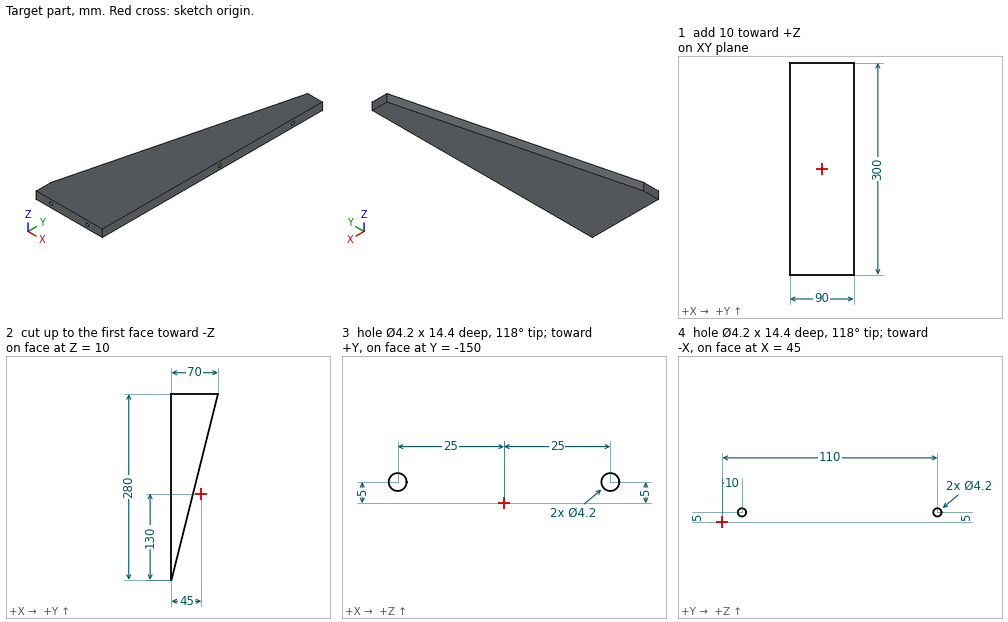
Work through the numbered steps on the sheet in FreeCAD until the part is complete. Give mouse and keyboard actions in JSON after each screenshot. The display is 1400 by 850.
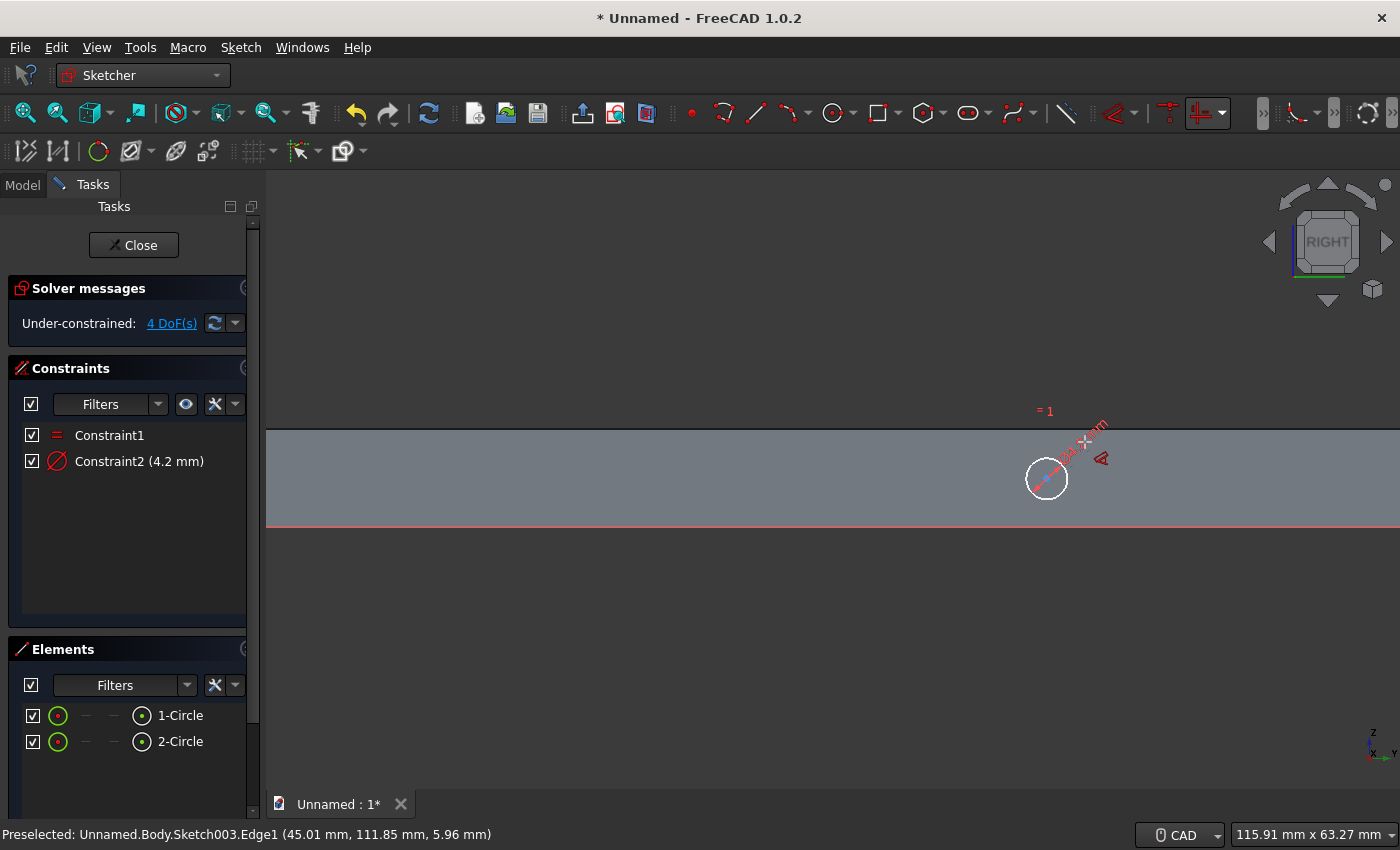
{"action": "left_click", "coordinate": [1047, 479]}
{"action": "left_click", "coordinate": [1081, 503]}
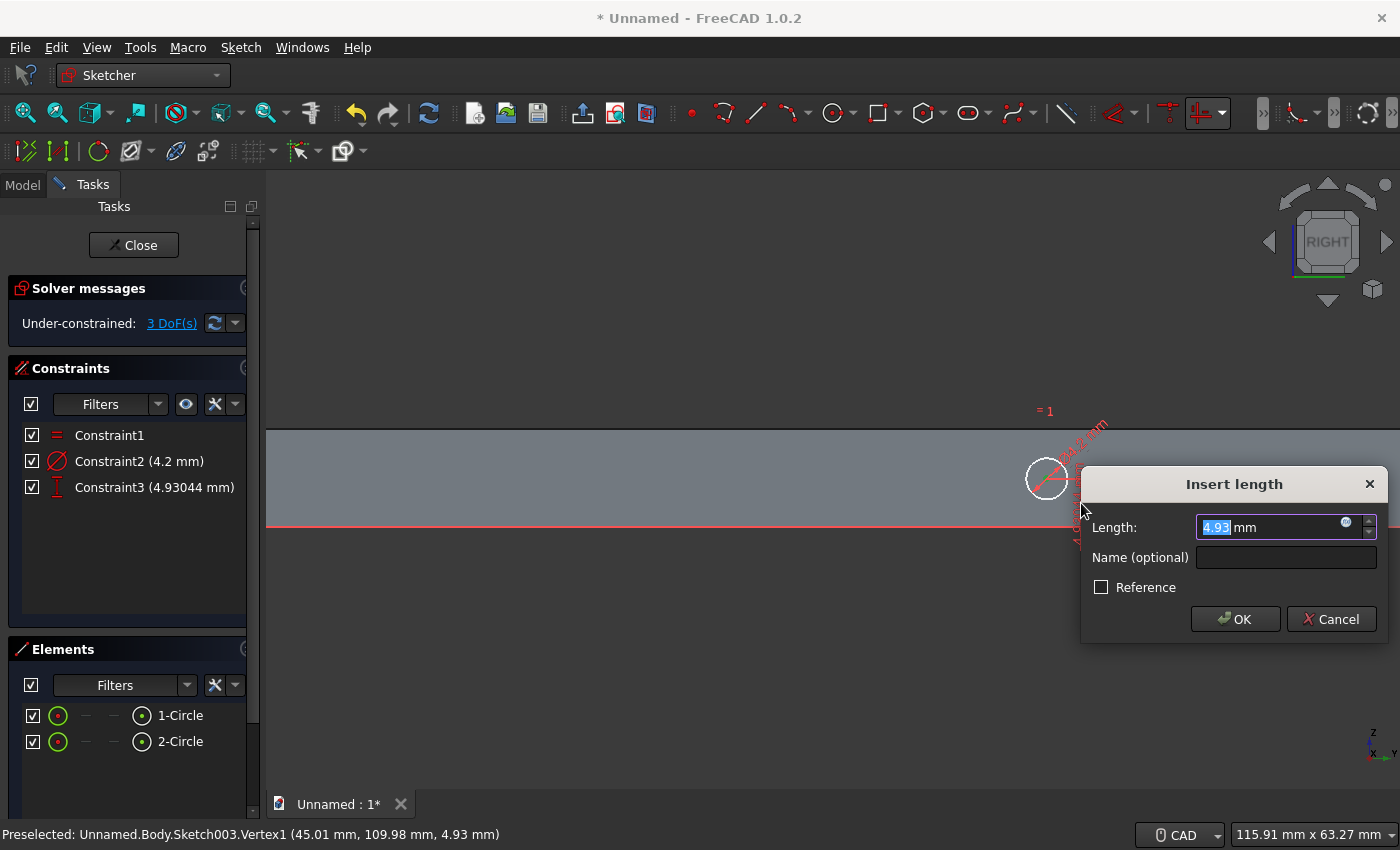
{"action": "type", "text": "5"}
{"action": "key", "text": "Return"}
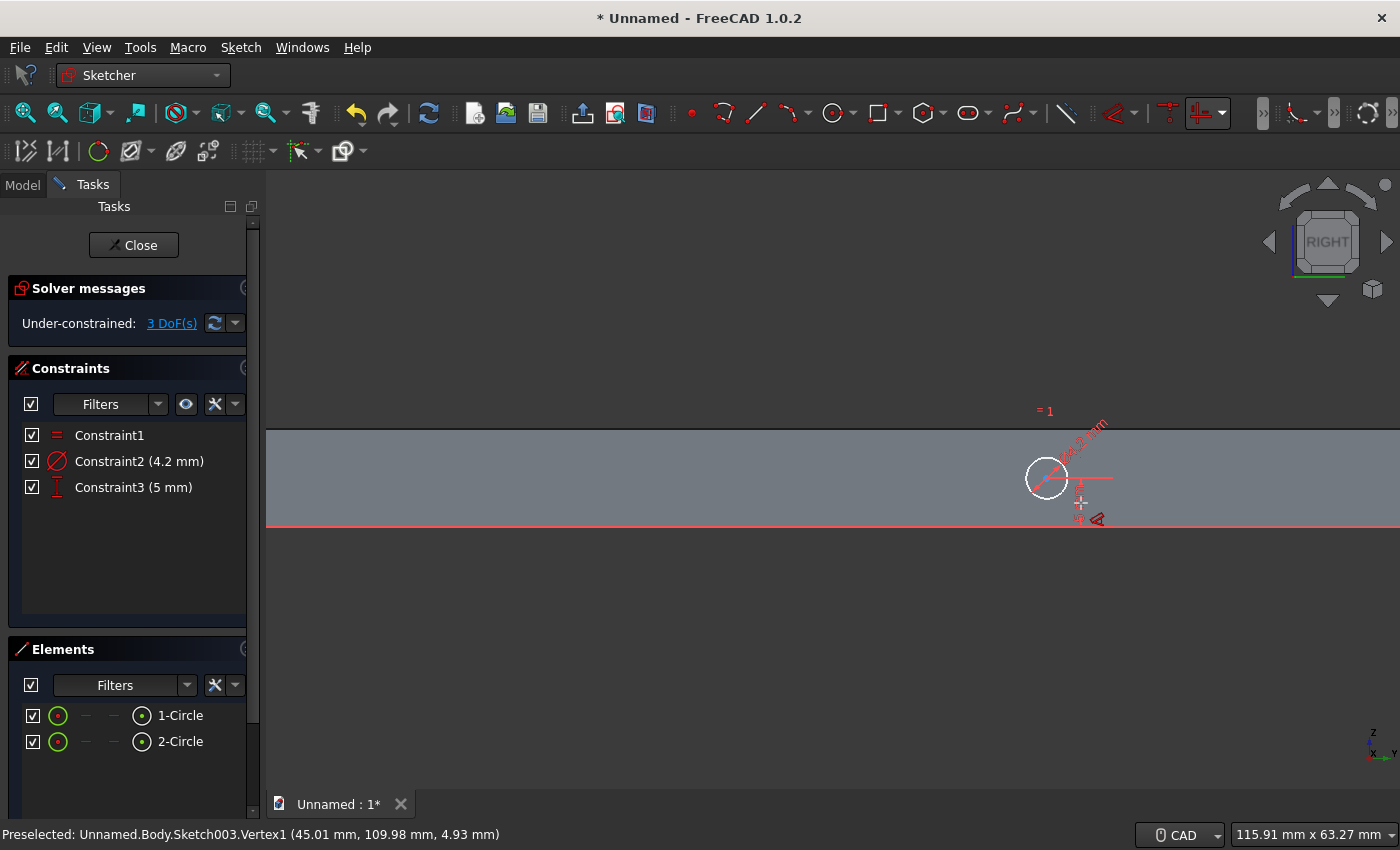
{"action": "scroll", "coordinate": [1063, 464], "scroll_direction": "down", "scroll_amount": 3}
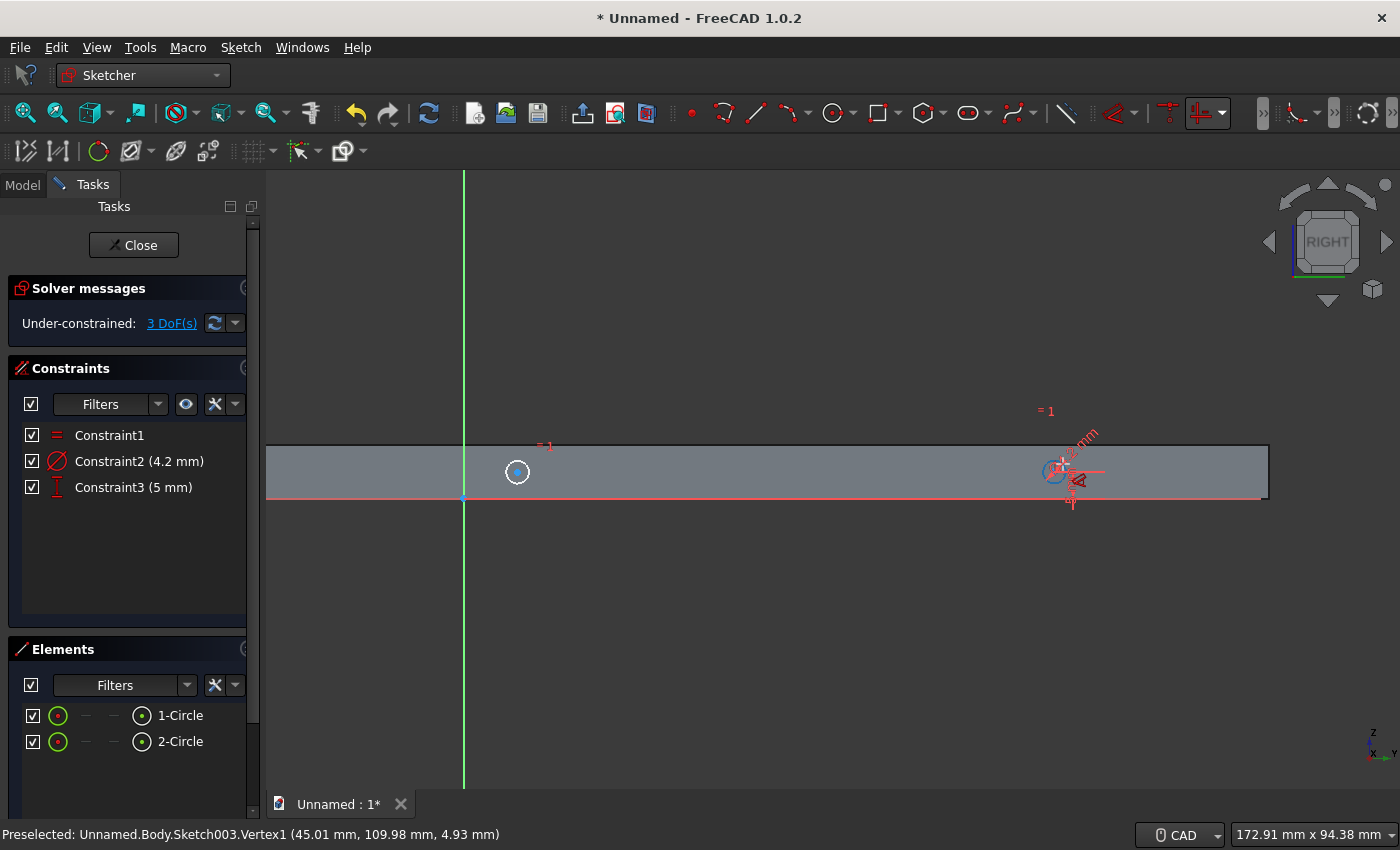
{"action": "scroll", "coordinate": [518, 472], "scroll_direction": "up", "scroll_amount": 2}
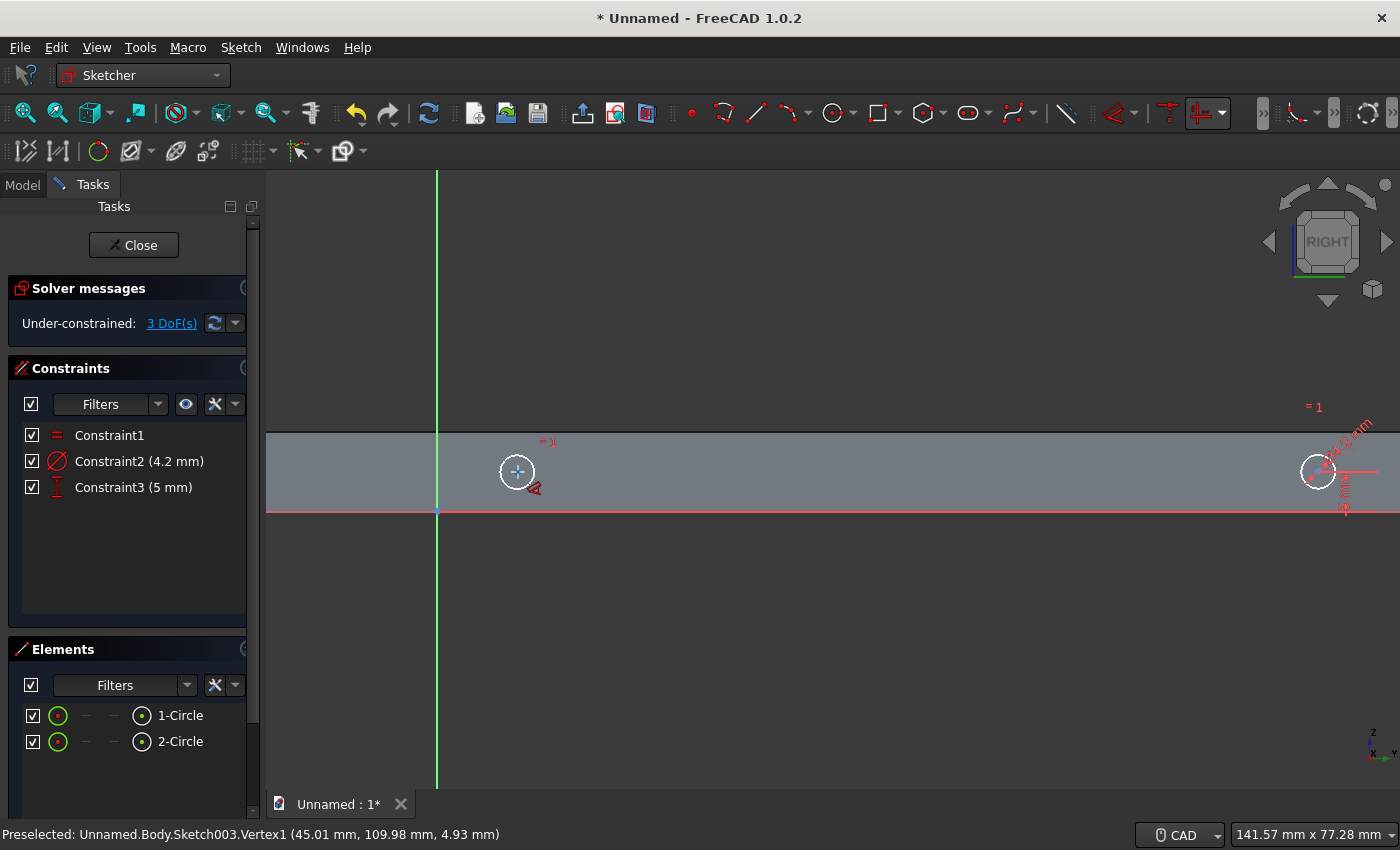
{"action": "left_click", "coordinate": [517, 472]}
{"action": "left_click", "coordinate": [403, 492]}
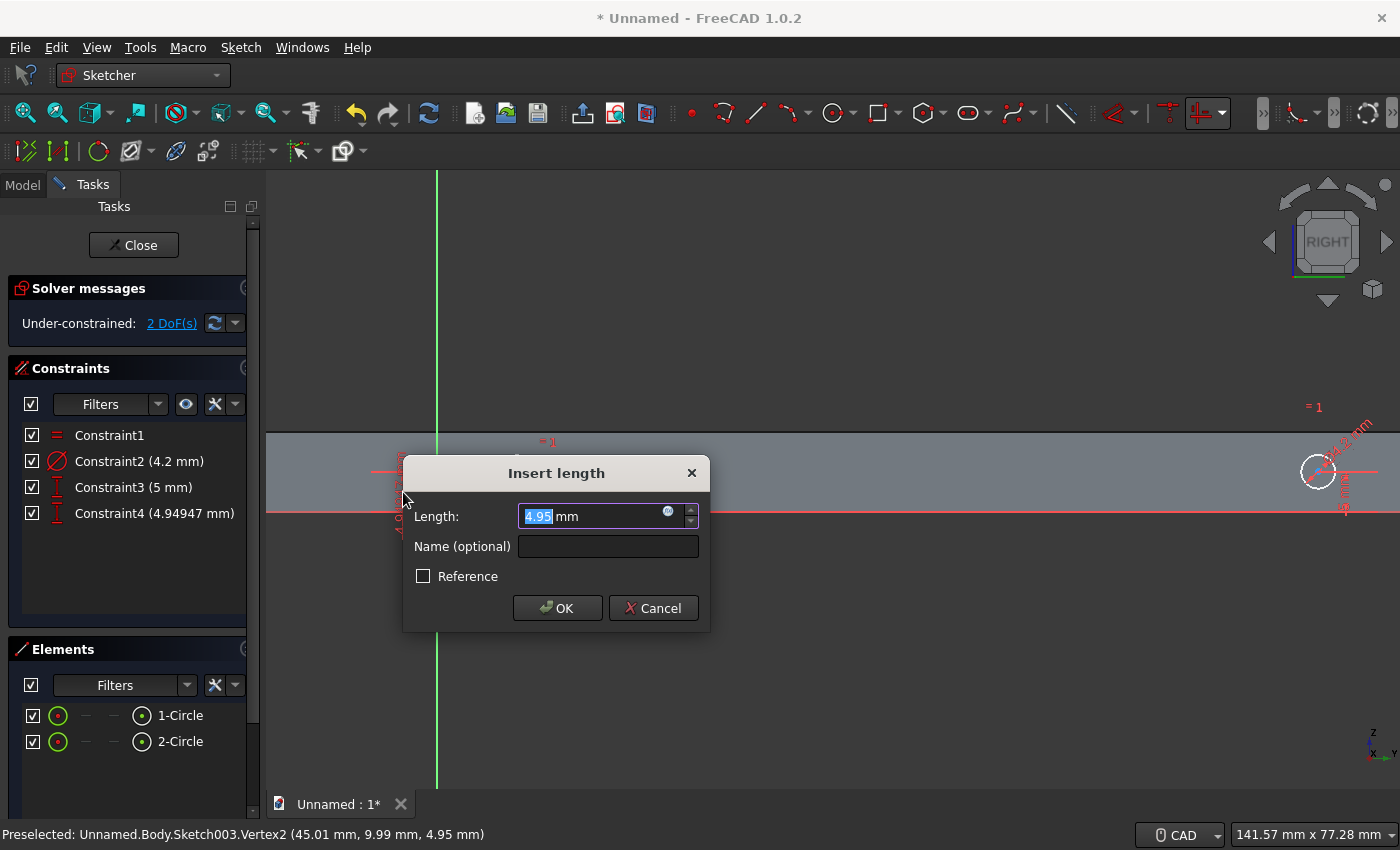
{"action": "type", "text": "5"}
{"action": "key", "text": "Return"}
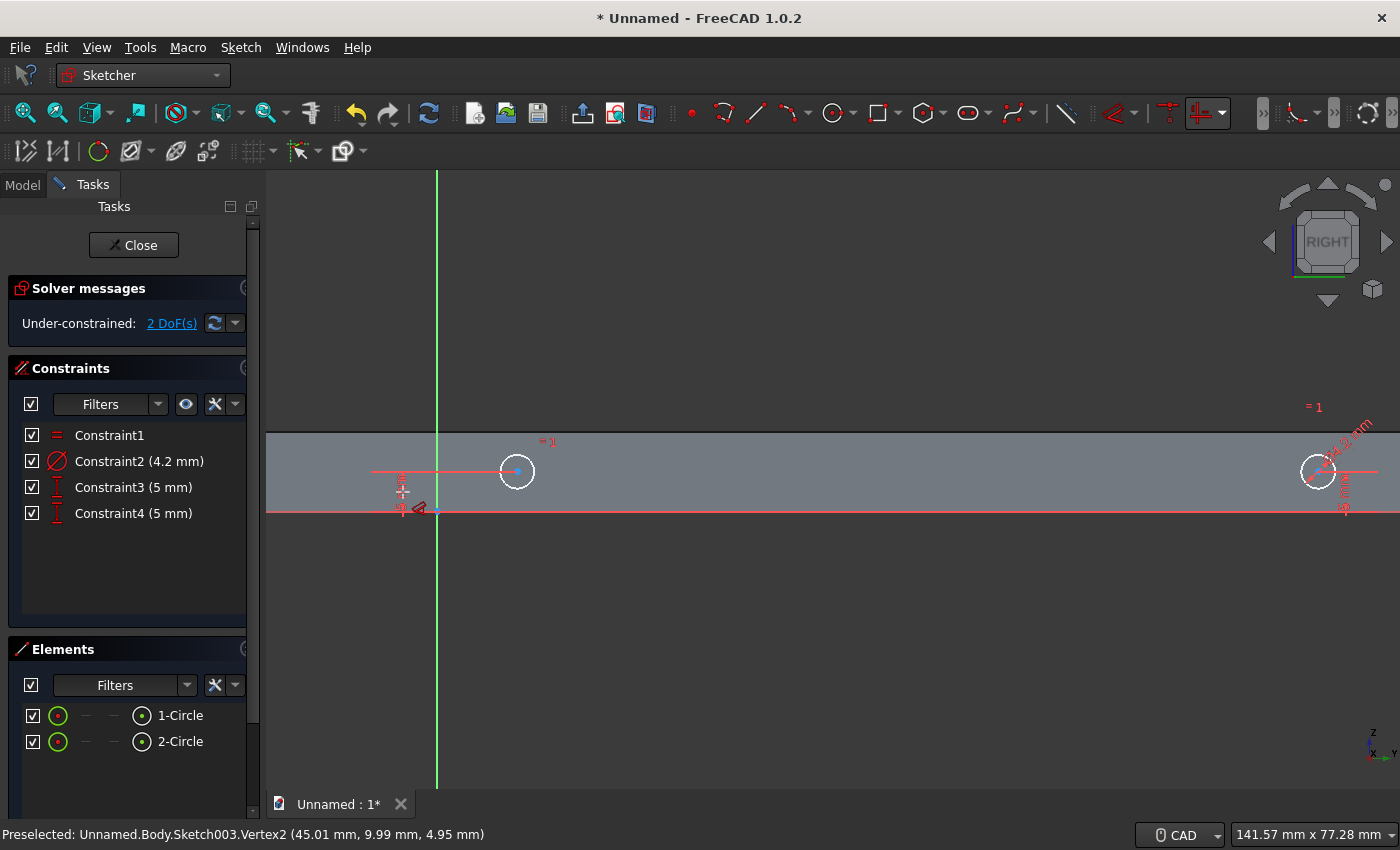
{"action": "left_click", "coordinate": [517, 472]}
{"action": "left_click", "coordinate": [477, 546]}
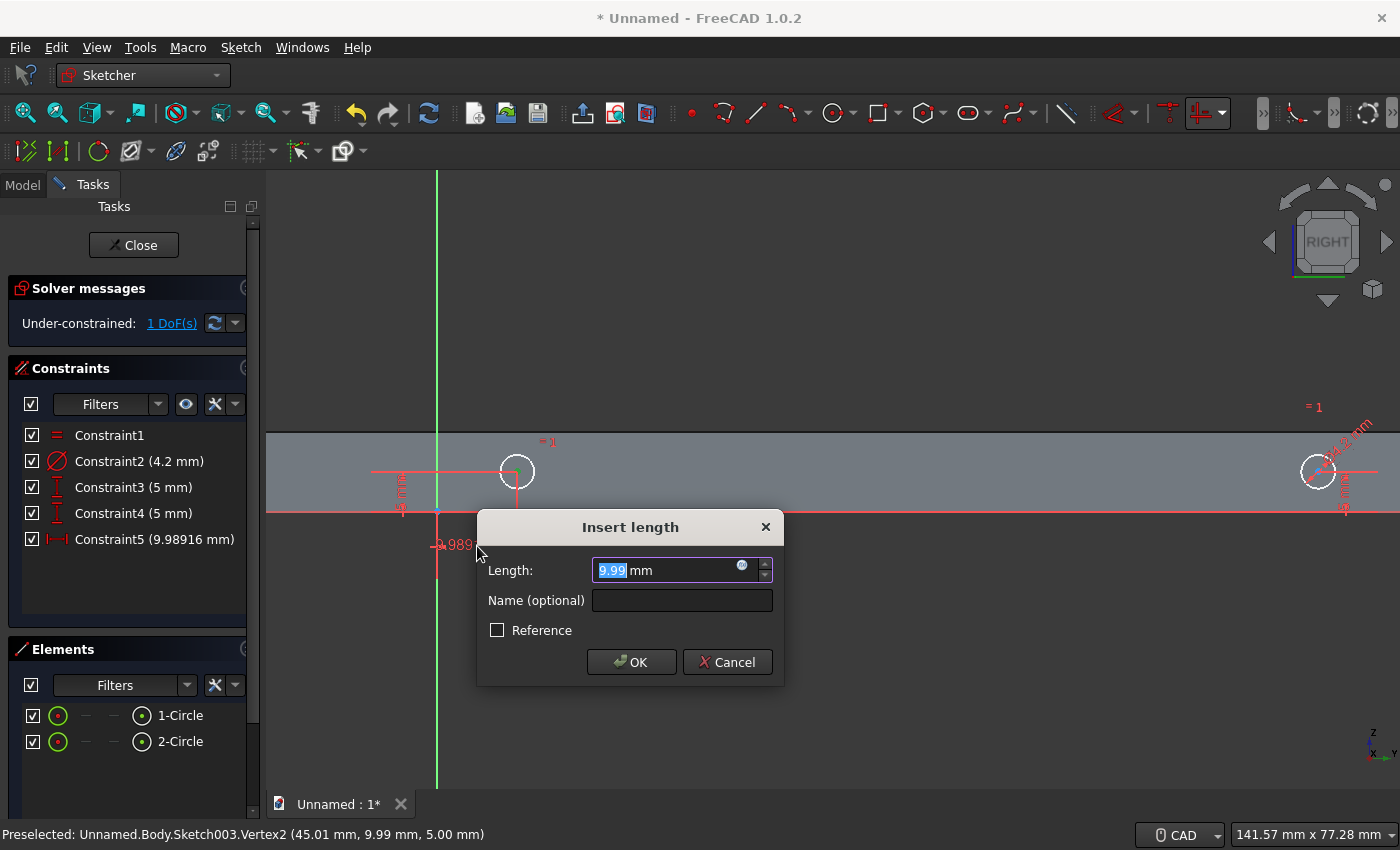
{"action": "type", "text": "10"}
{"action": "key", "text": "Return"}